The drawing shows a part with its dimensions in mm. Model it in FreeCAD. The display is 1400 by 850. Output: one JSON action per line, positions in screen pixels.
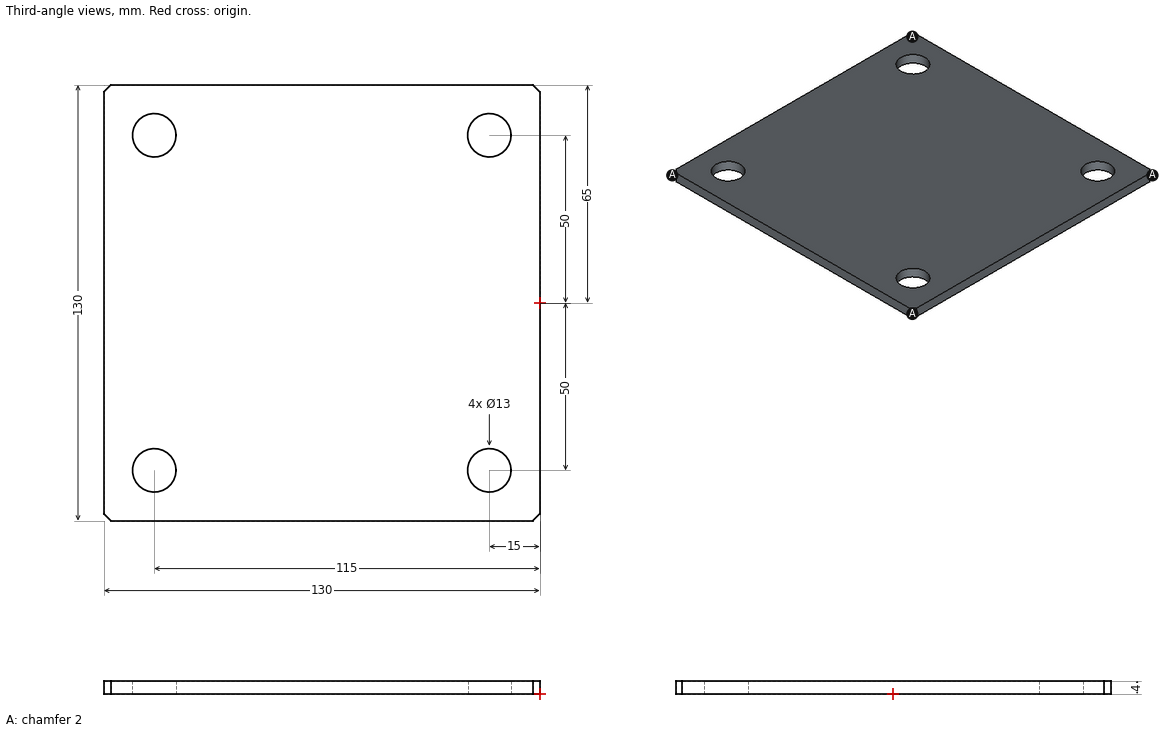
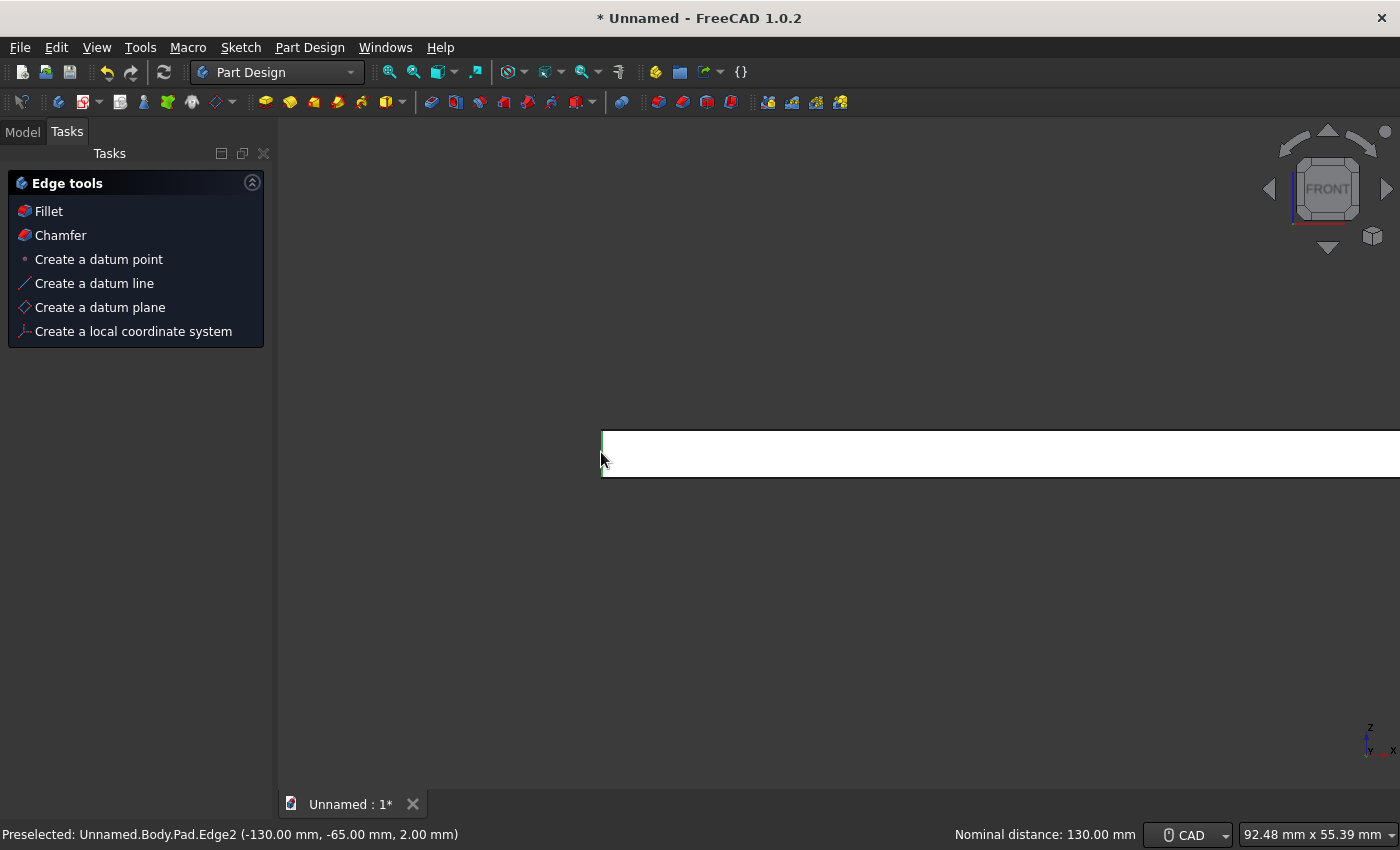
{"action": "left_click", "coordinate": [390, 72]}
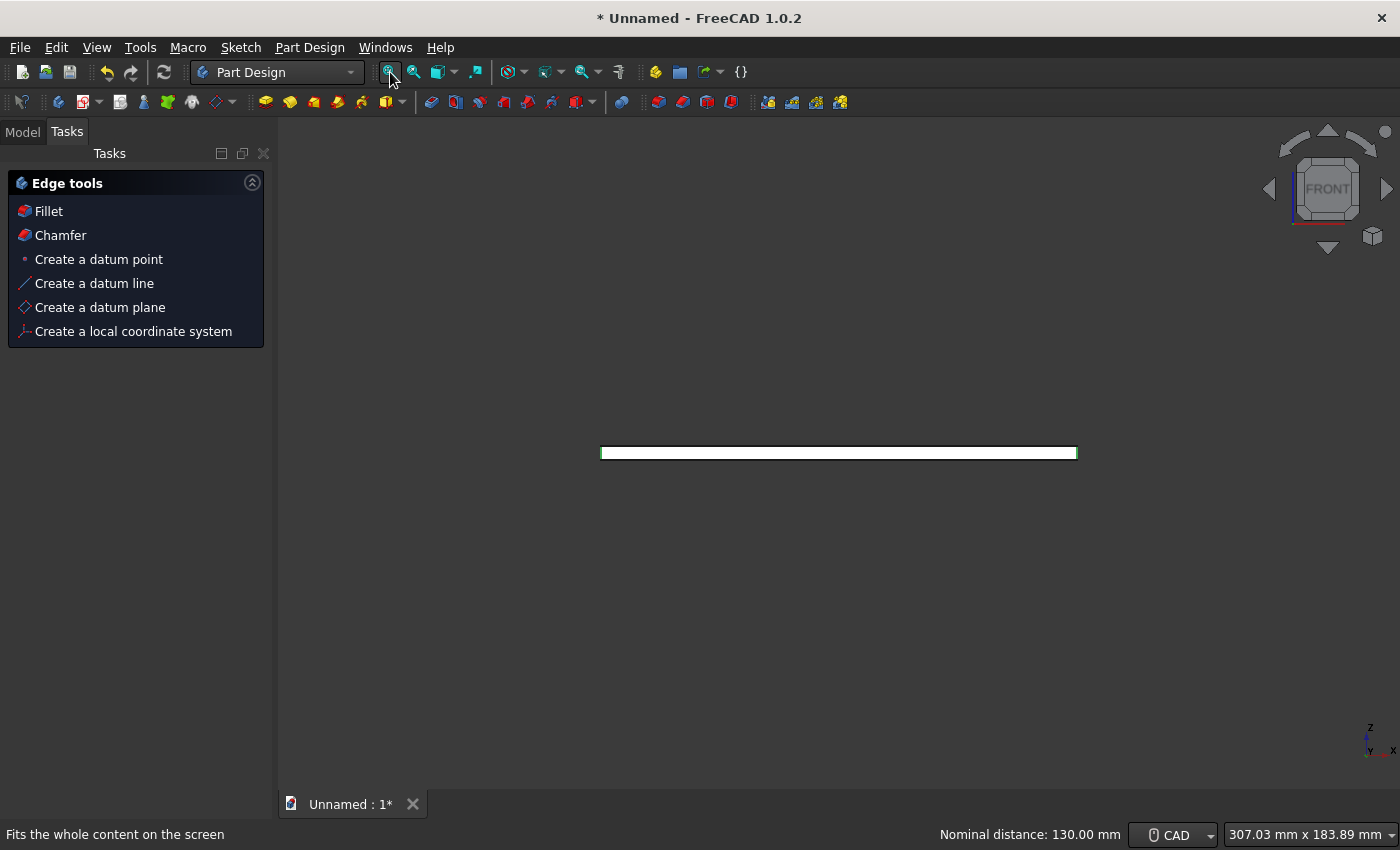
{"action": "key", "text": "3"}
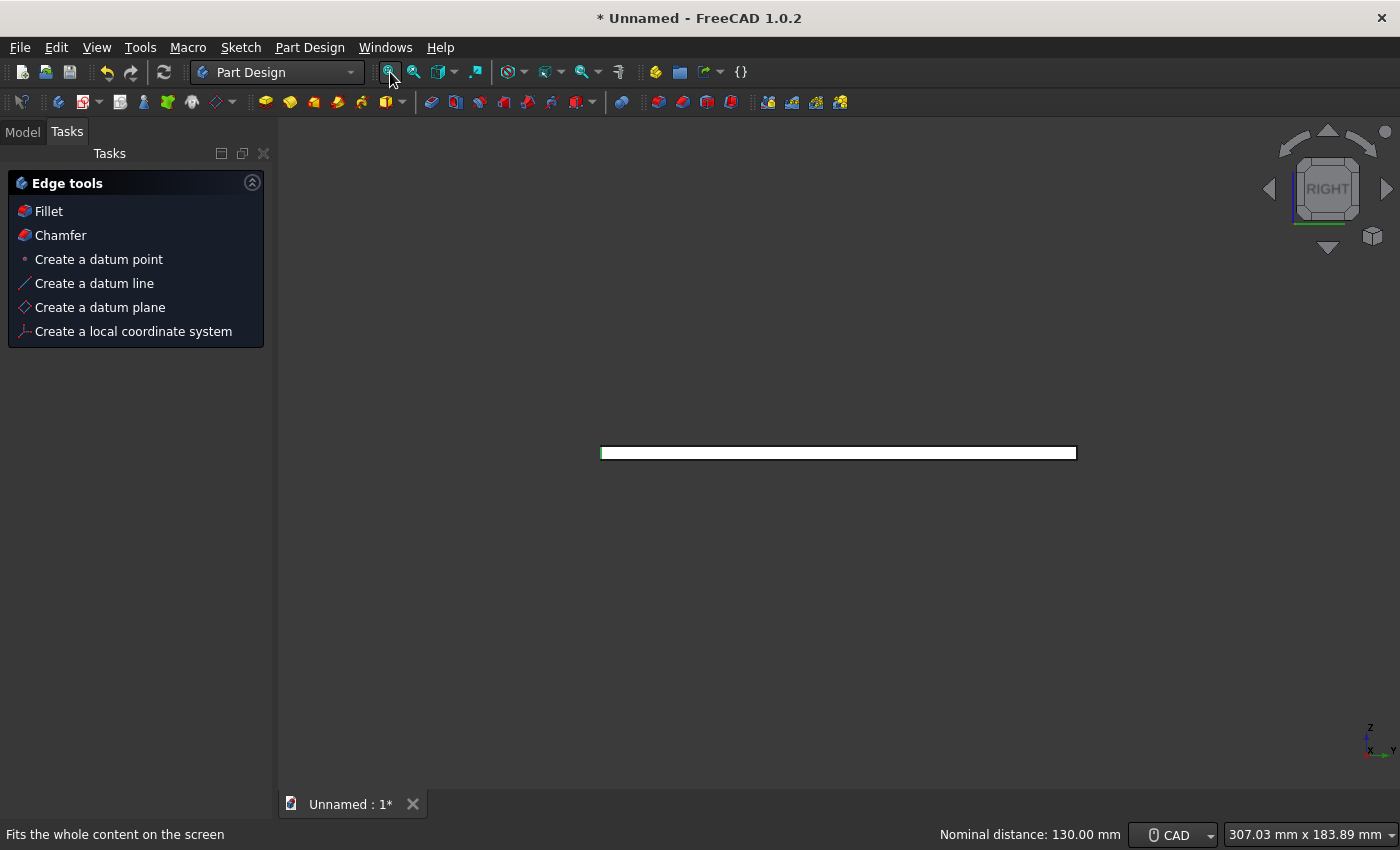
{"action": "left_click", "coordinate": [390, 72]}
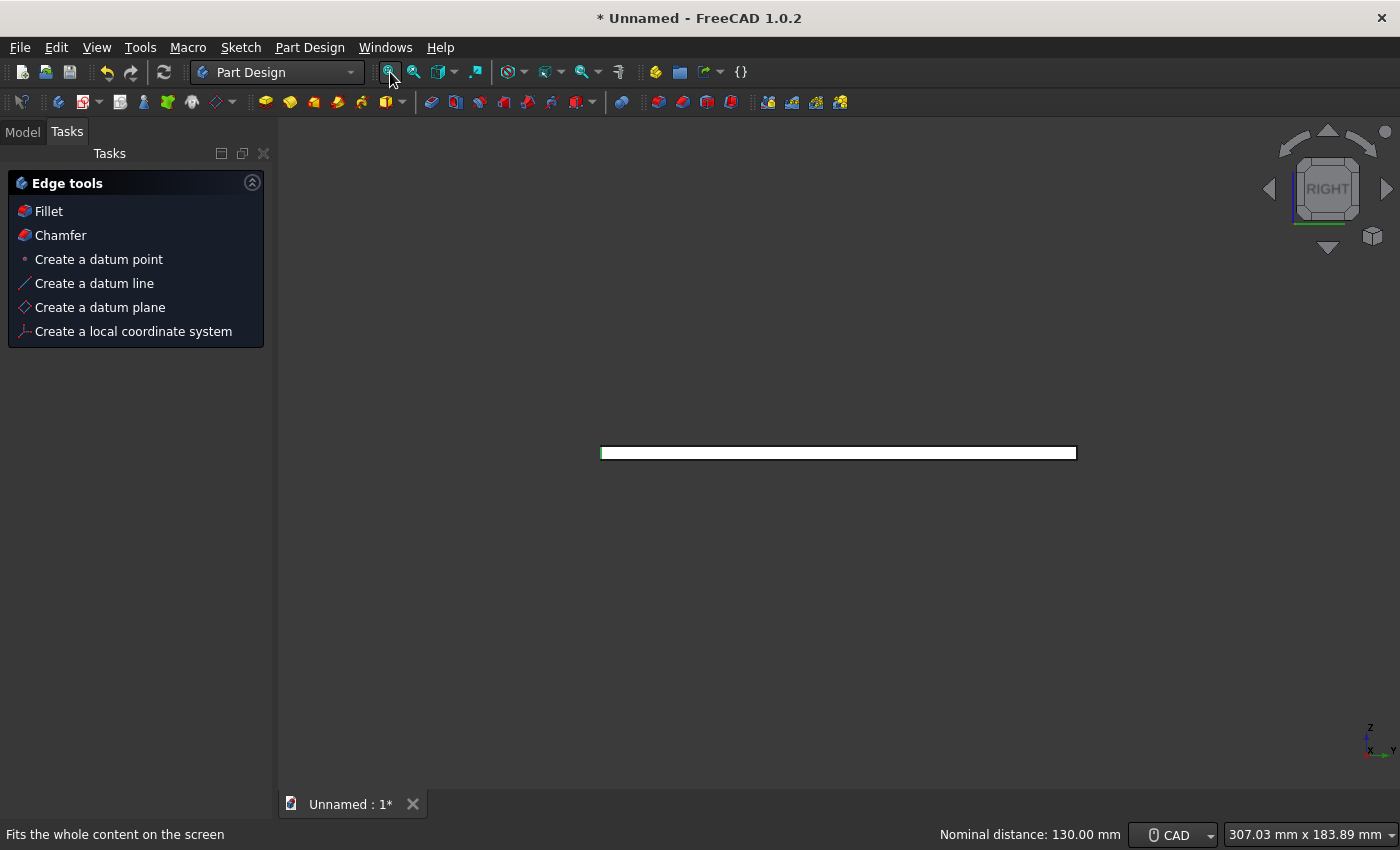
{"action": "left_click", "coordinate": [1077, 452], "text": "ctrl"}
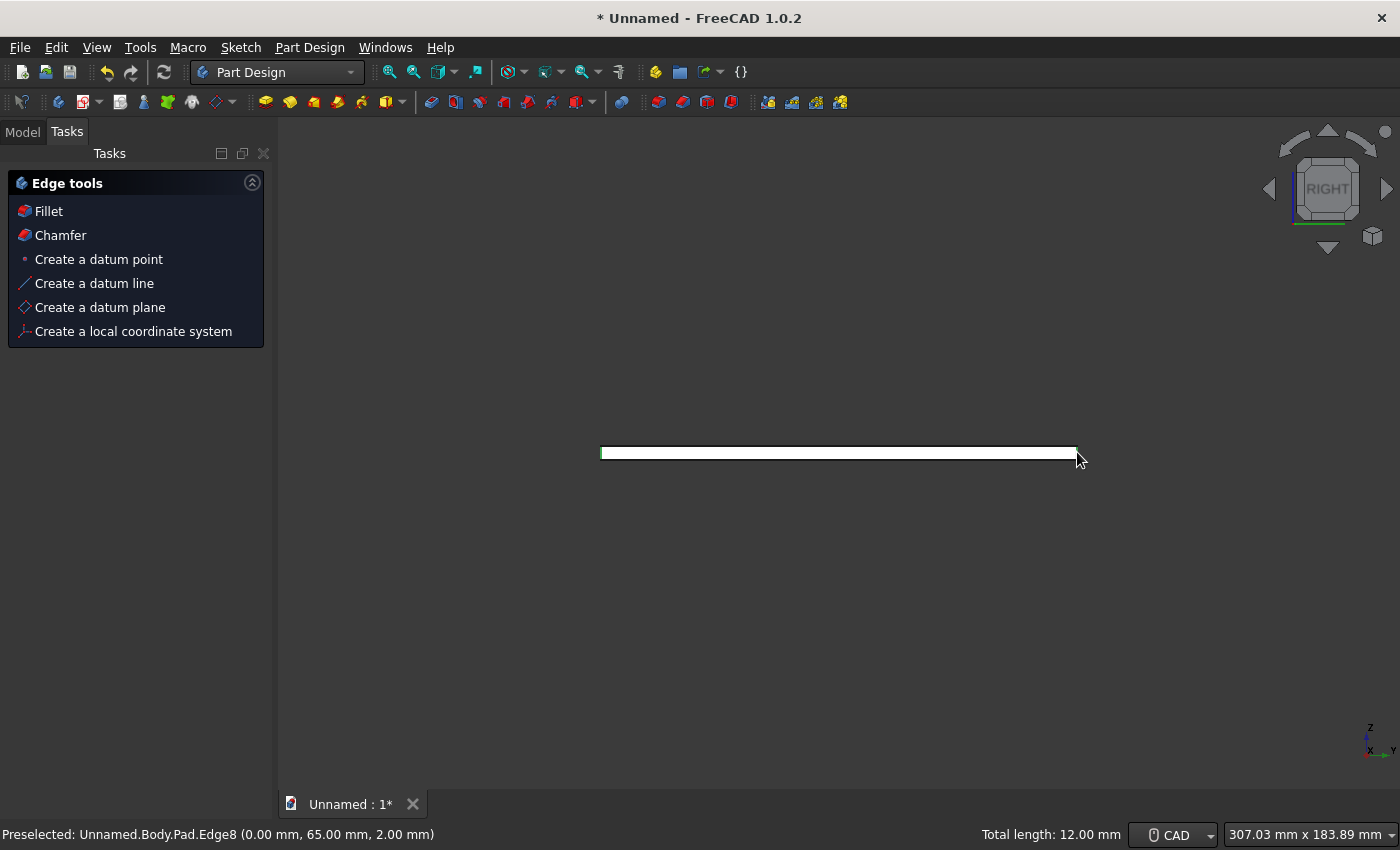
{"action": "scroll", "coordinate": [1077, 452], "scroll_direction": "up", "scroll_amount": 6}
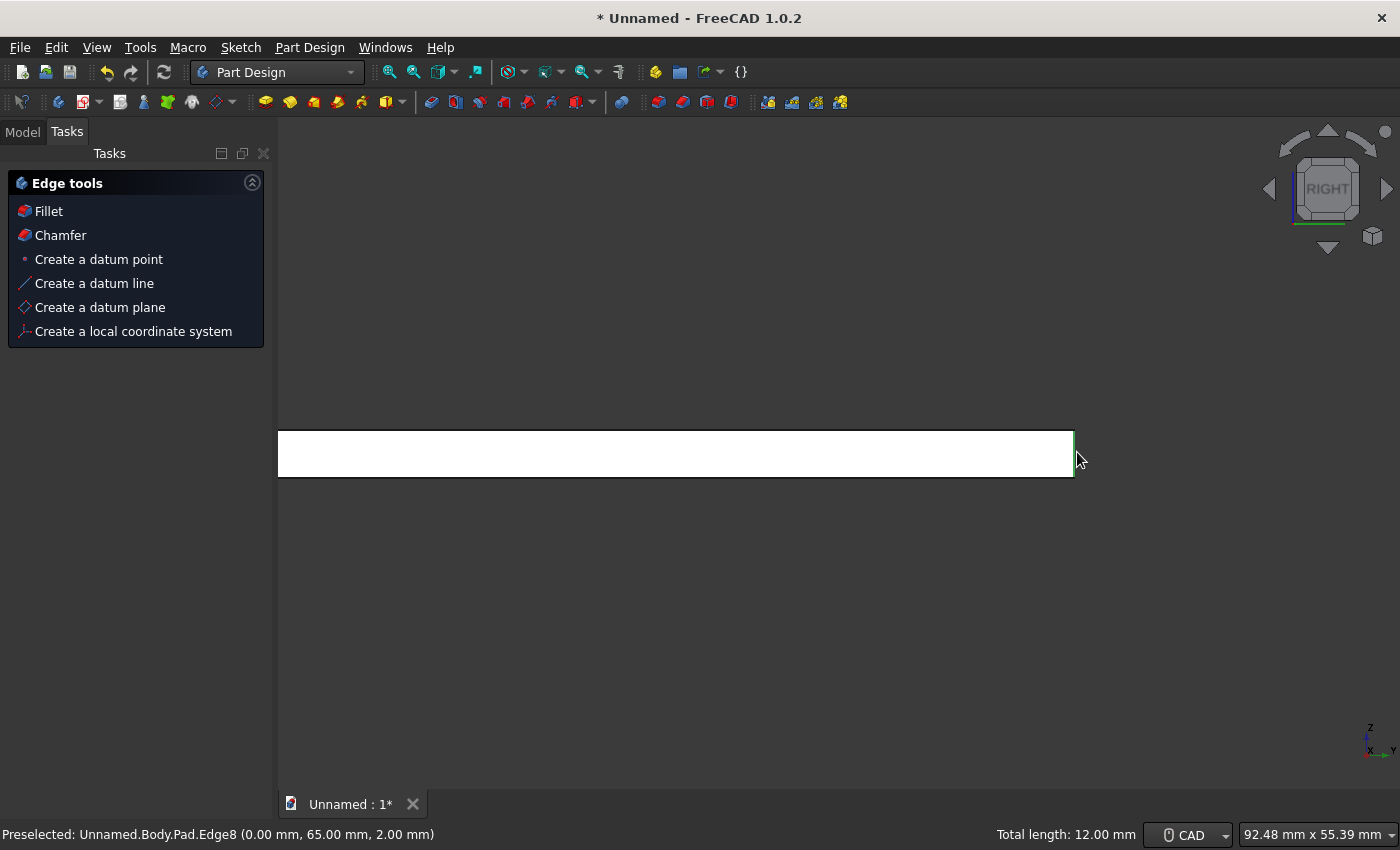
{"action": "left_click", "coordinate": [390, 72]}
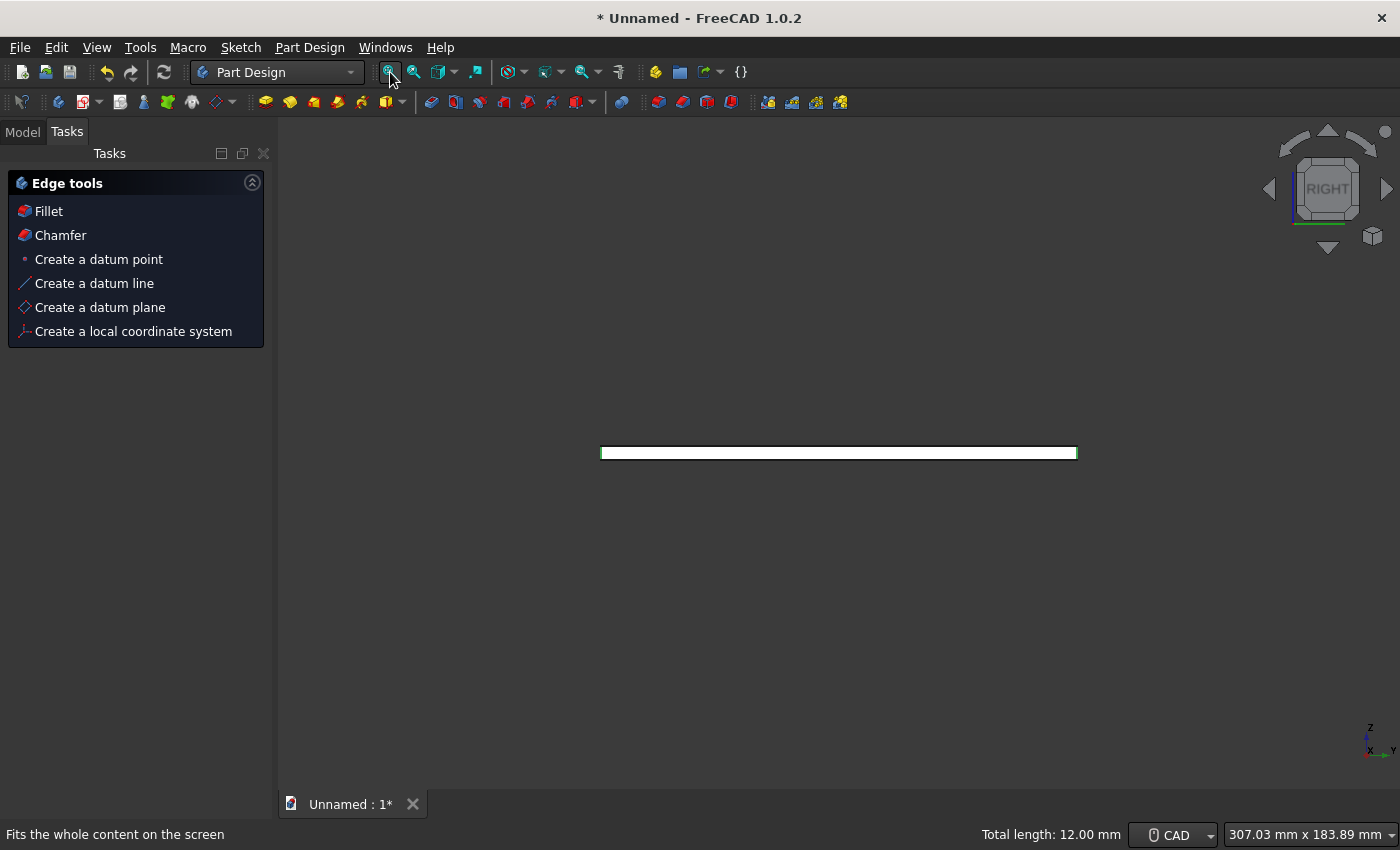
{"action": "key", "text": "5"}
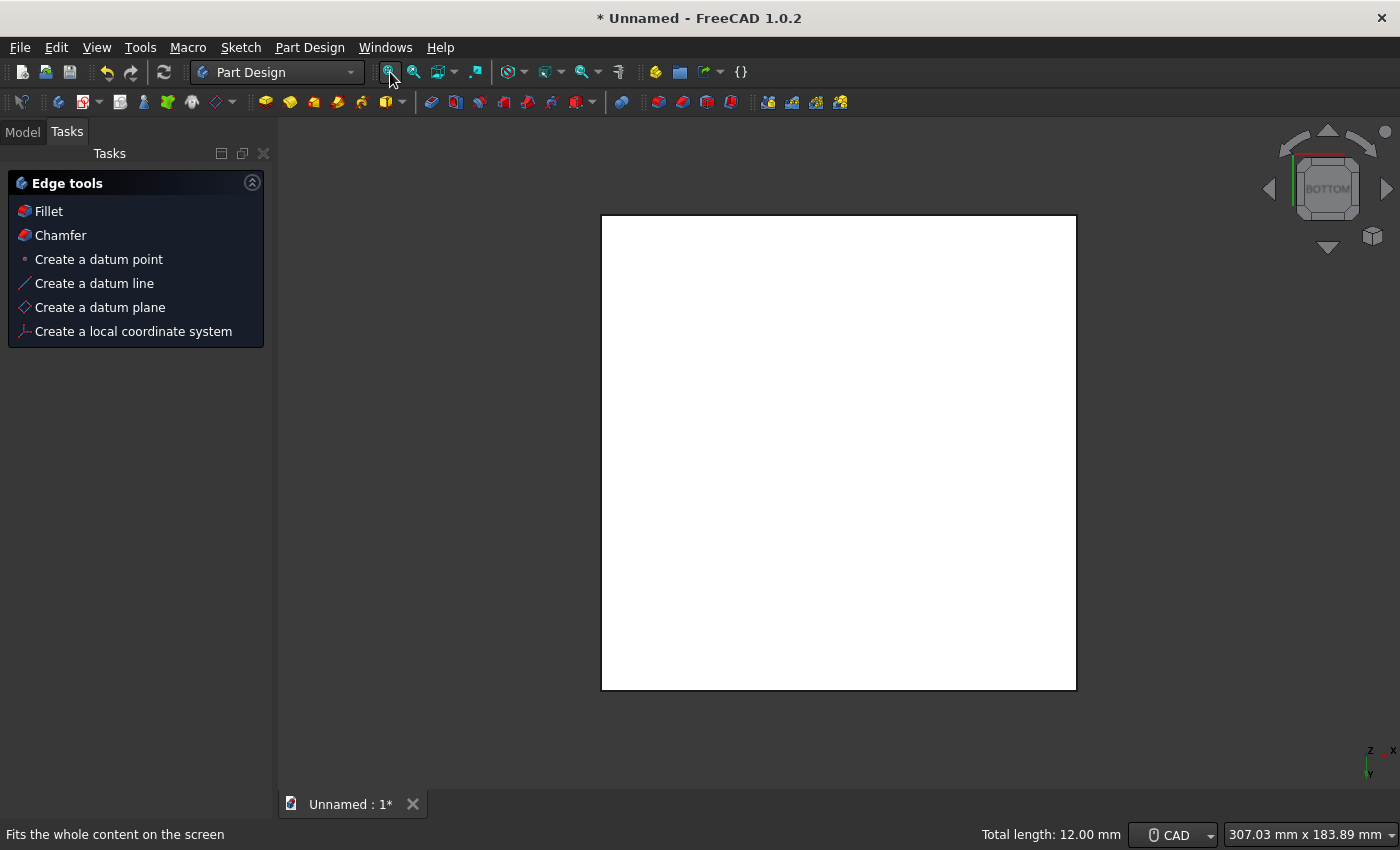
{"action": "scroll", "coordinate": [601, 690], "scroll_direction": "up", "scroll_amount": 6}